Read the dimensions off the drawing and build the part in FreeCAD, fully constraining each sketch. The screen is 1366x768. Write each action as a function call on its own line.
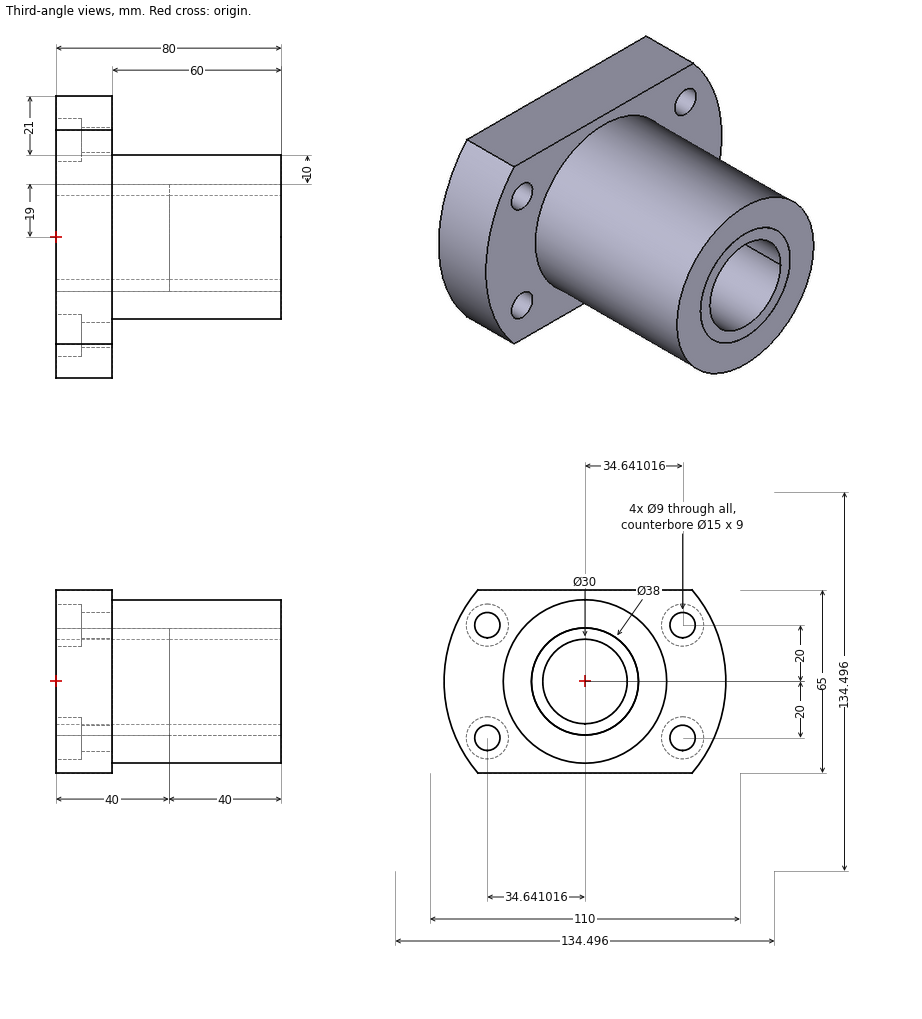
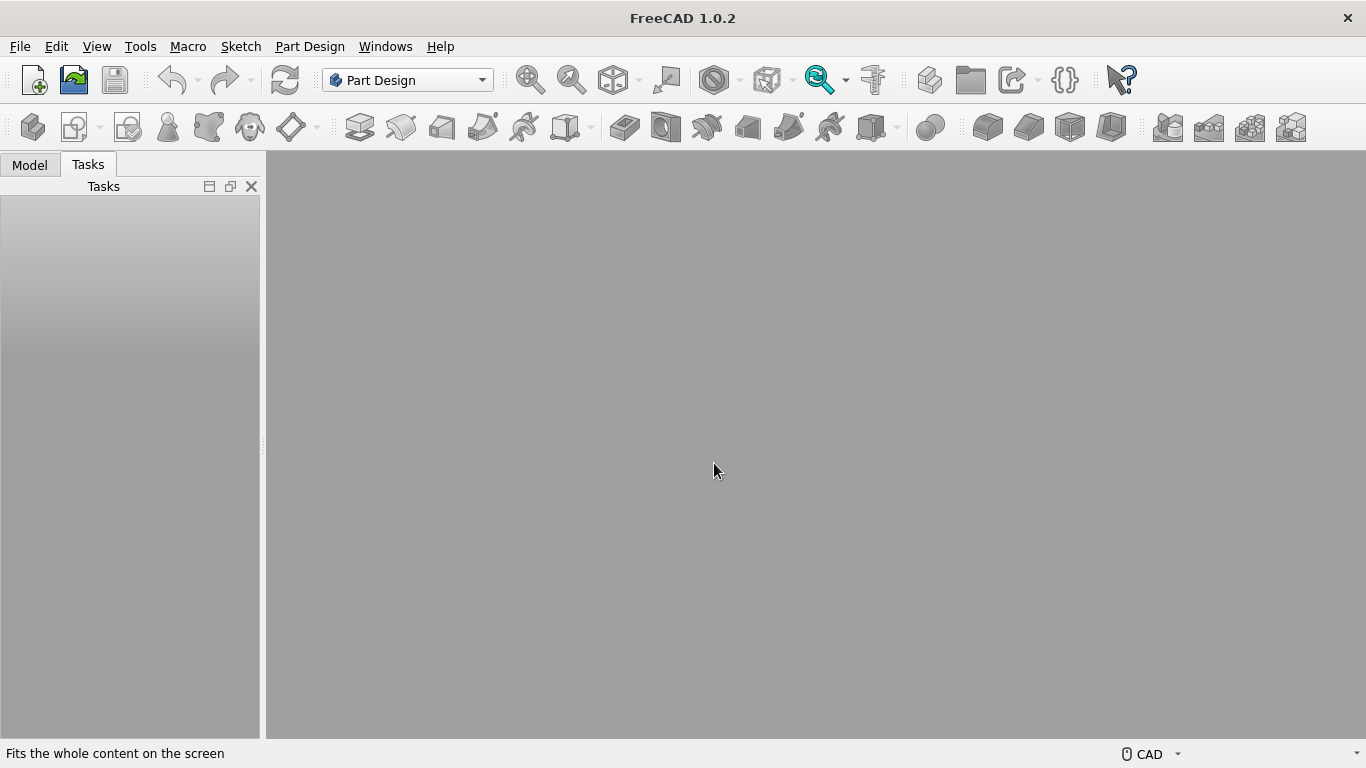
key(ctrl+n)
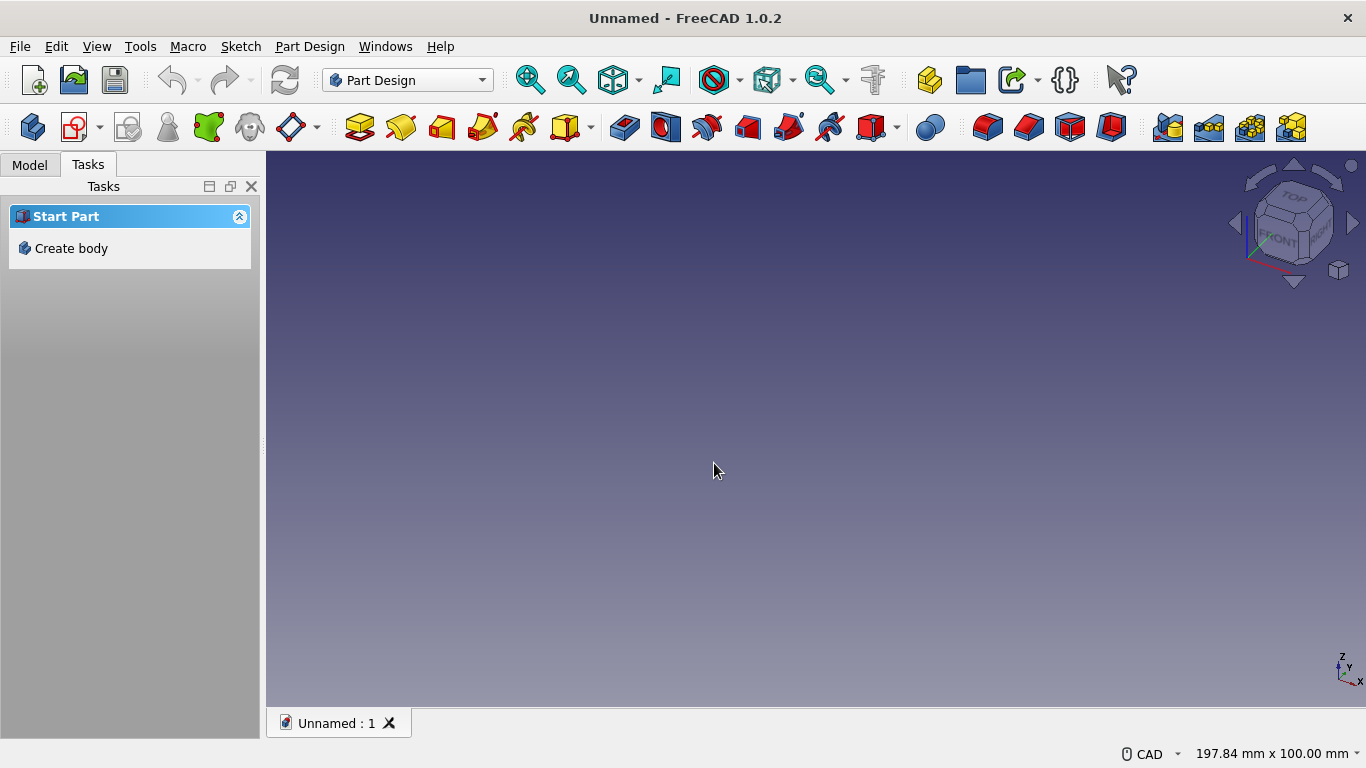
click(74, 128)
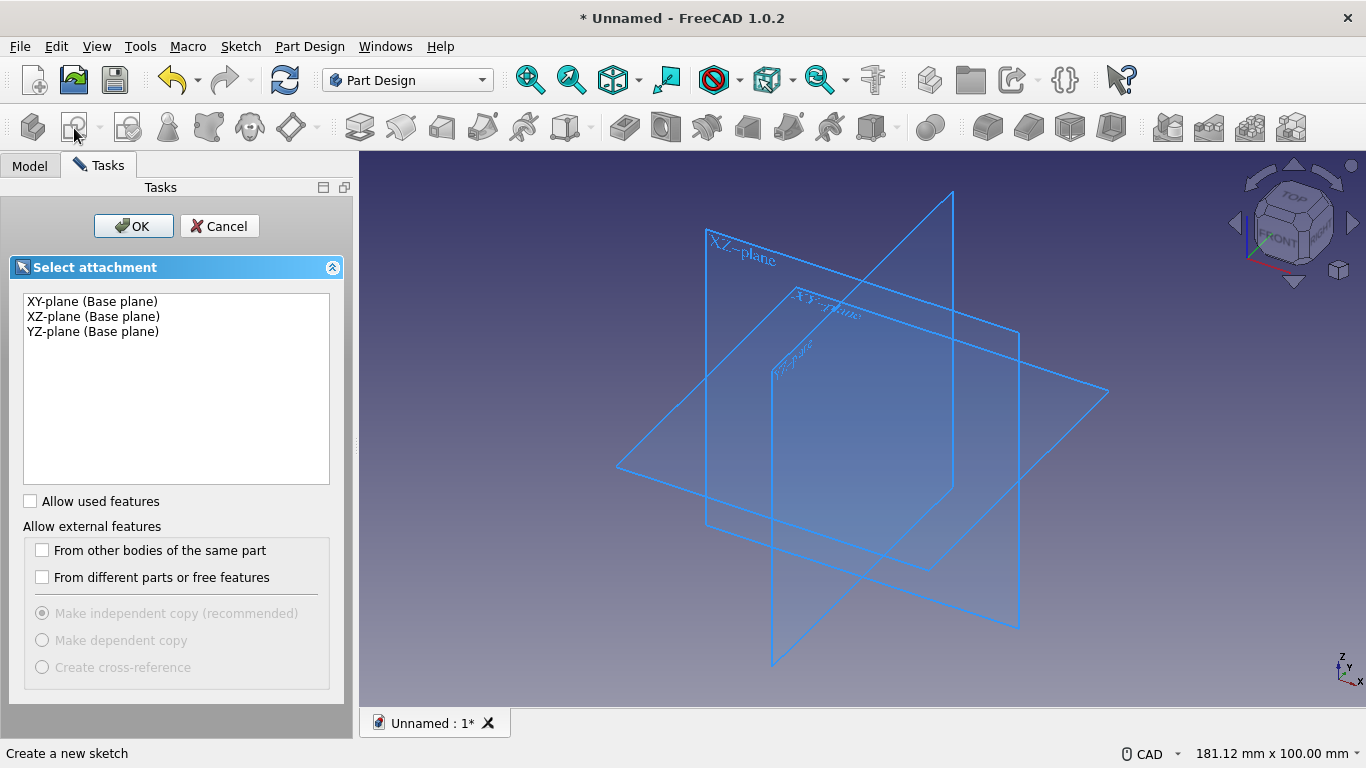
click(84, 302)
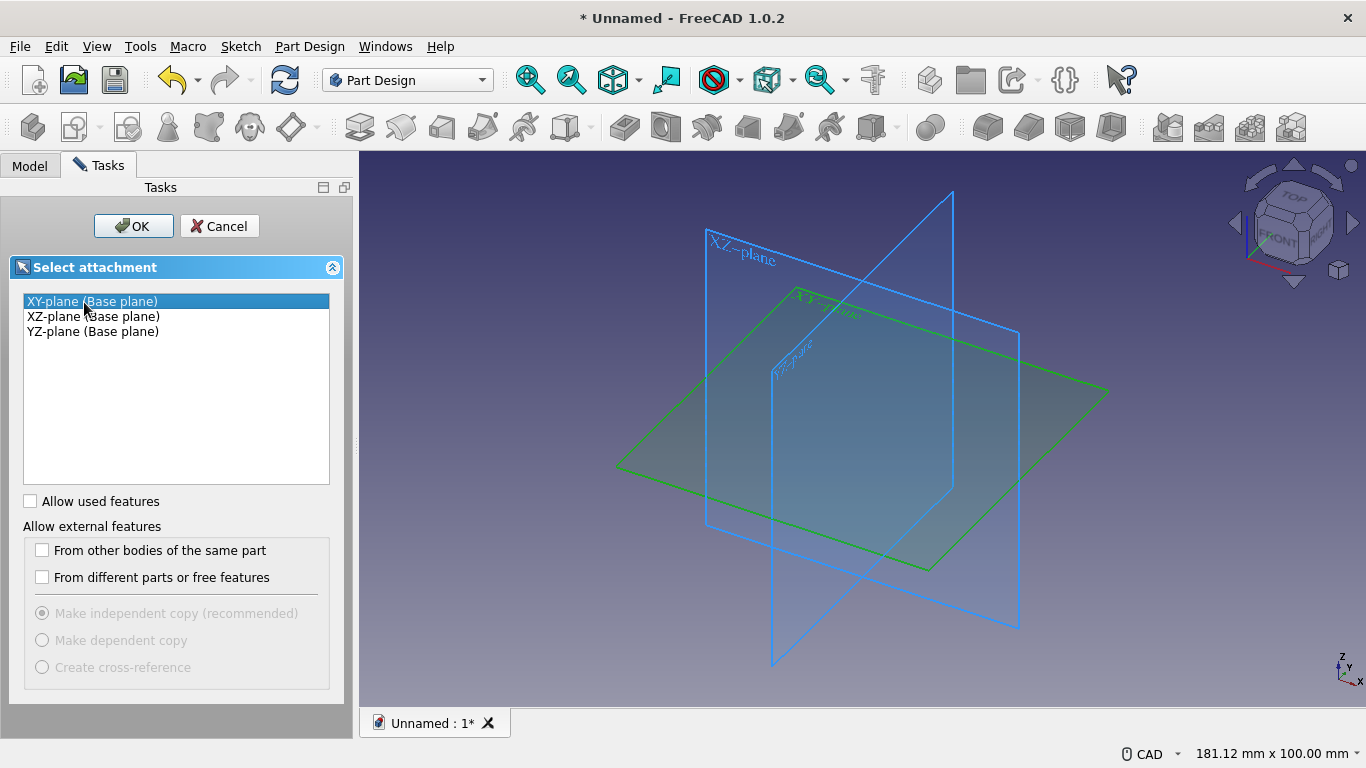
click(134, 226)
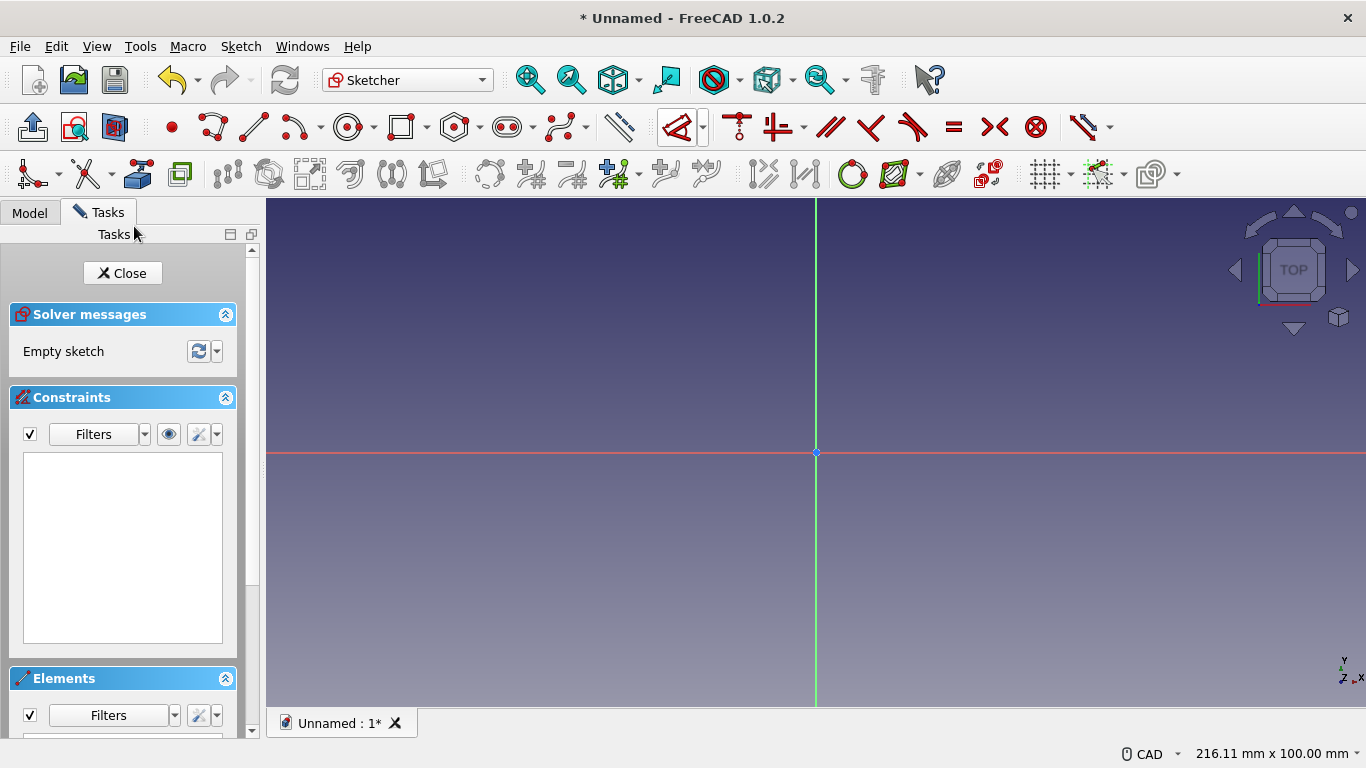
scroll(294, 679, down, 1)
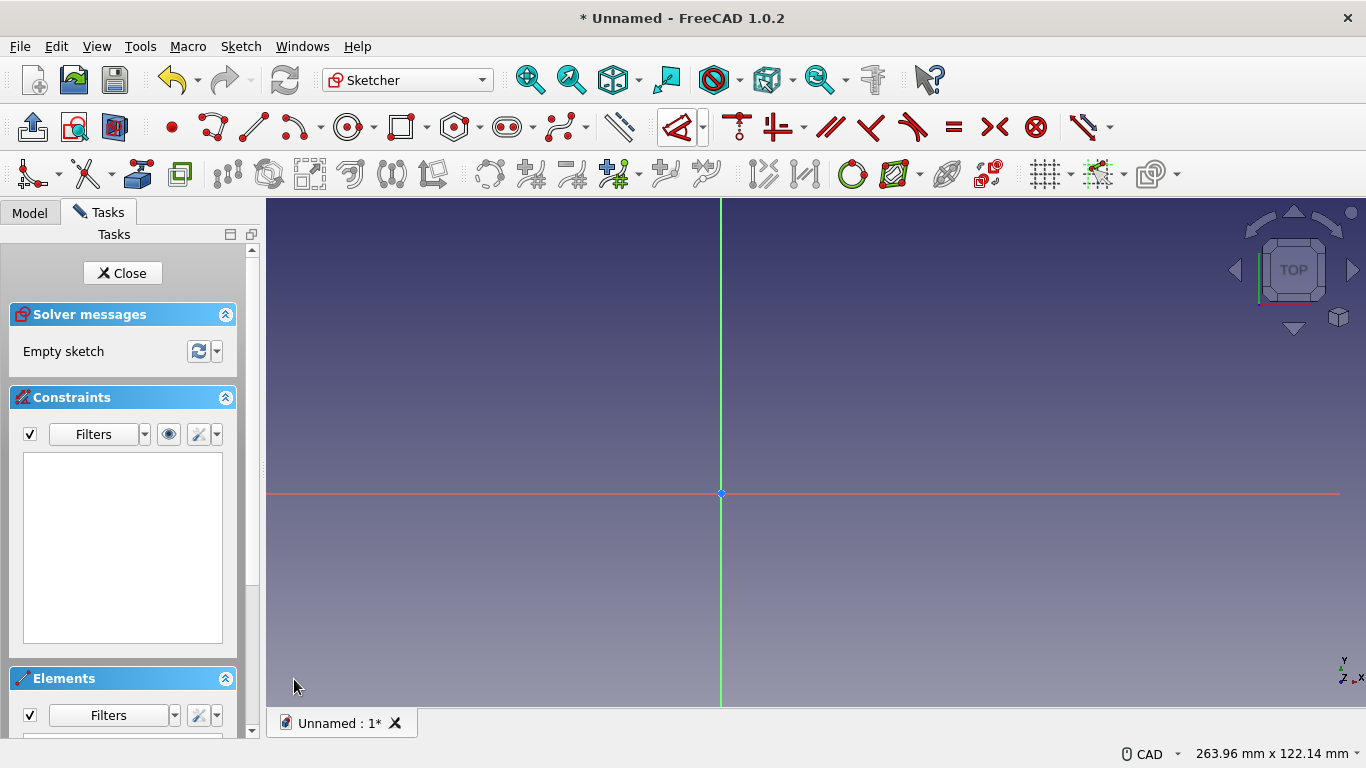
scroll(1174, 262, up, 2)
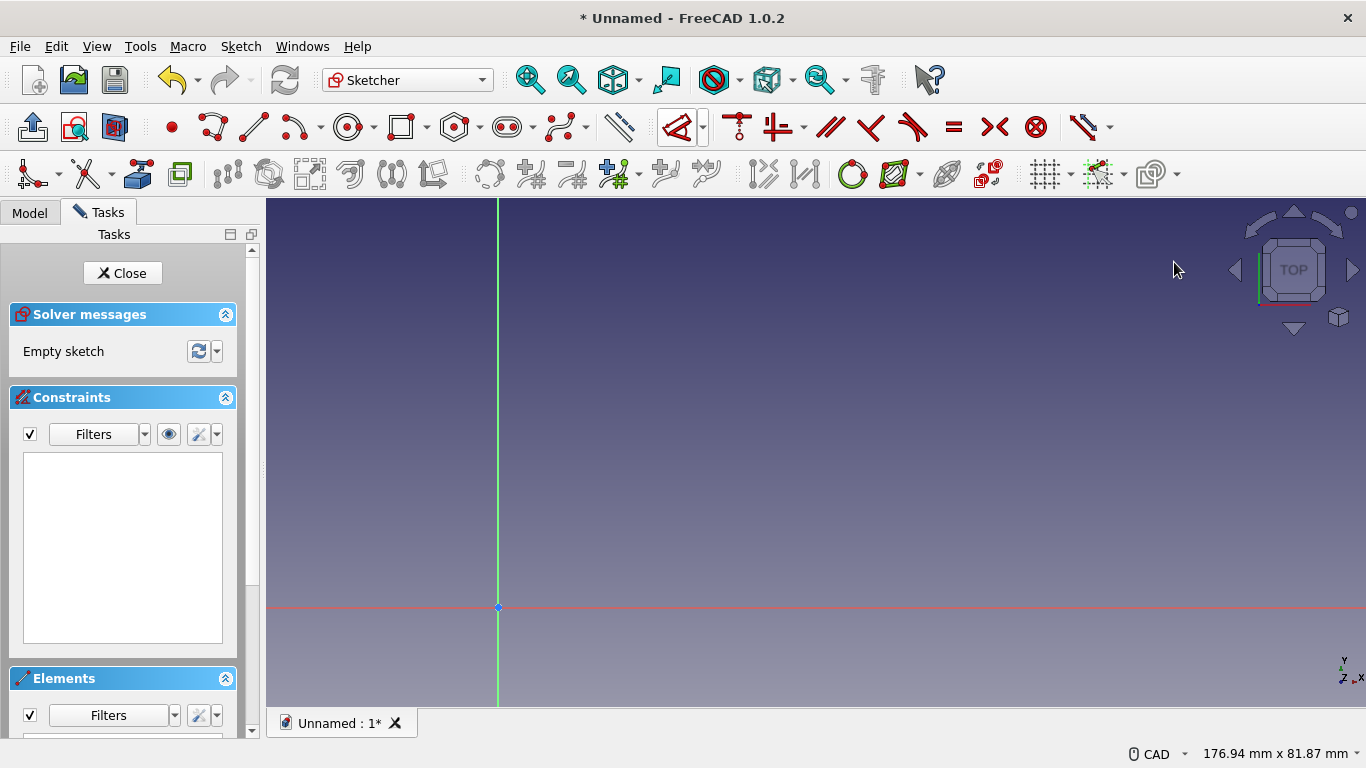
click(213, 128)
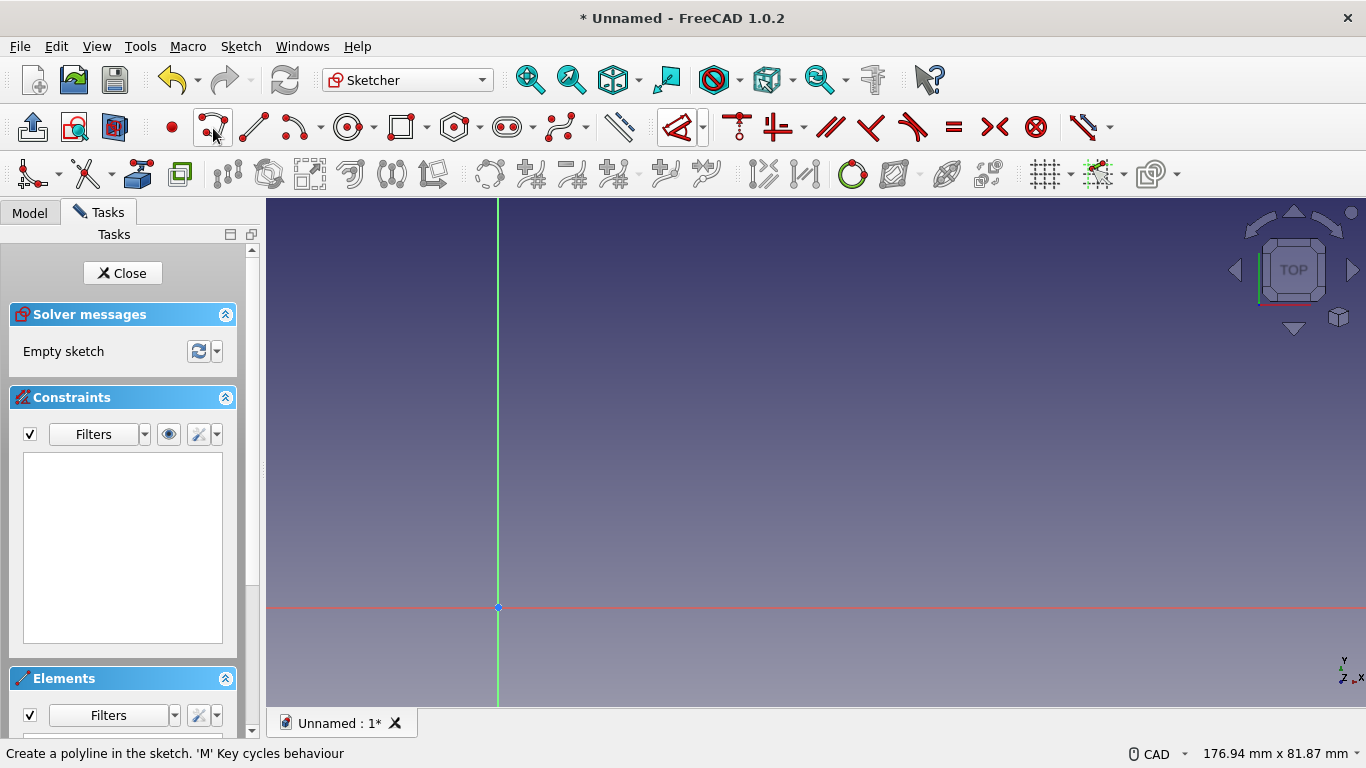
click(498, 490)
click(996, 490)
click(996, 427)
click(623, 427)
click(623, 297)
click(507, 297)
click(498, 491)
key(Escape)
key(Escape)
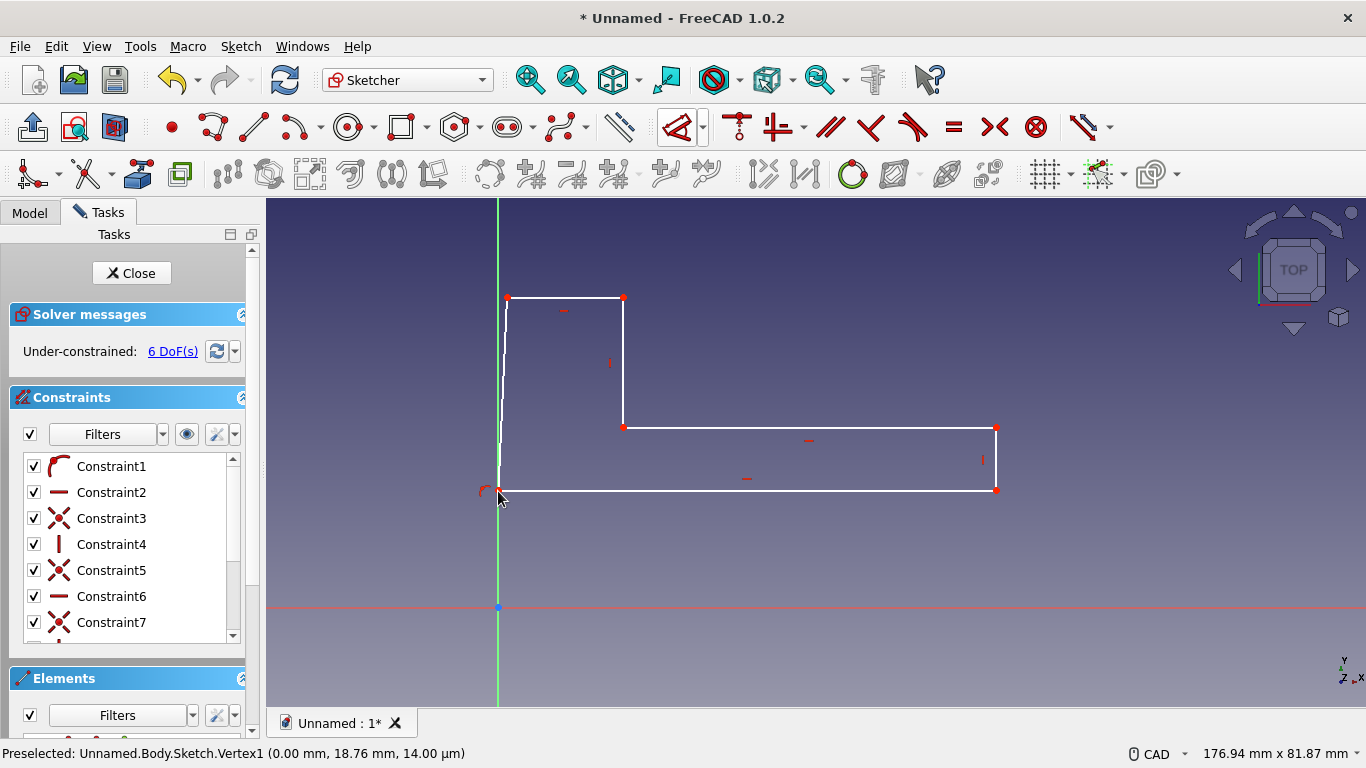
click(501, 433)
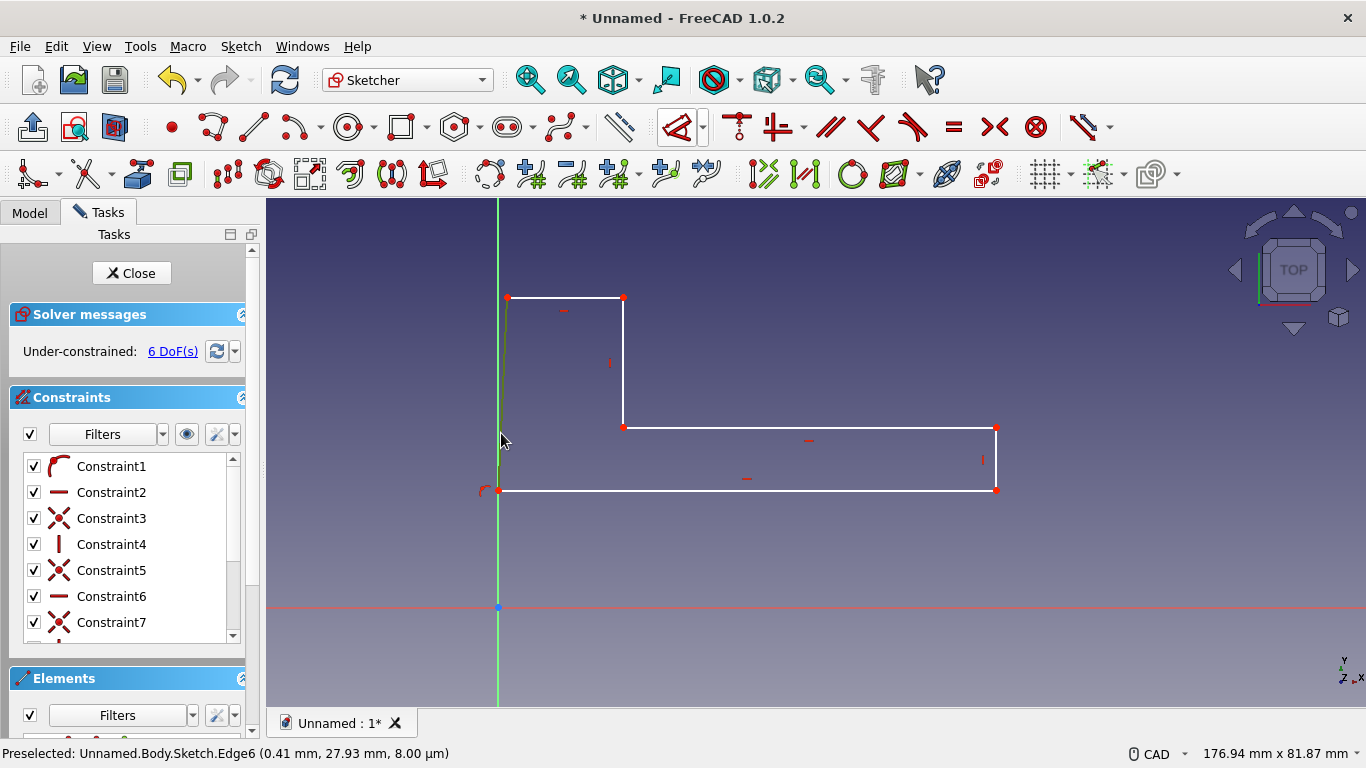
key(v)